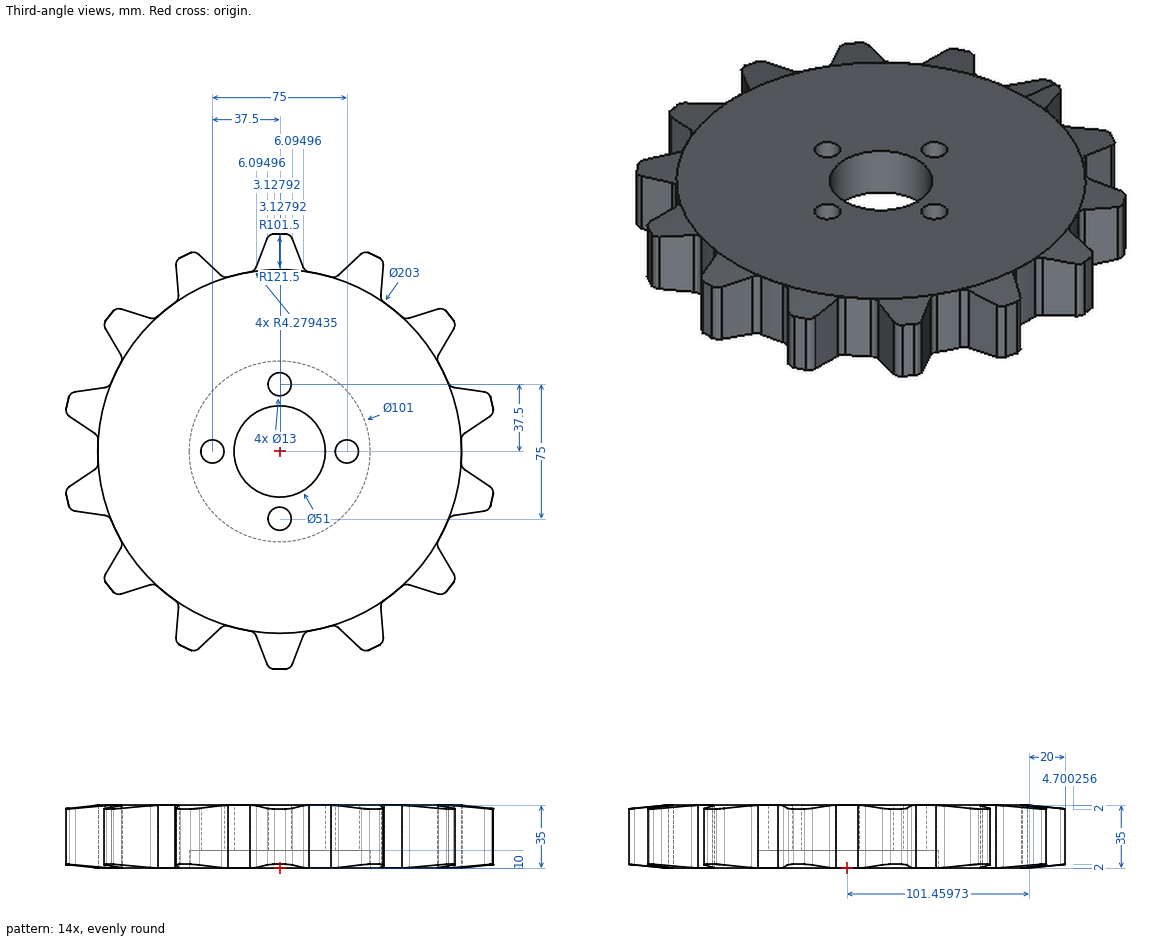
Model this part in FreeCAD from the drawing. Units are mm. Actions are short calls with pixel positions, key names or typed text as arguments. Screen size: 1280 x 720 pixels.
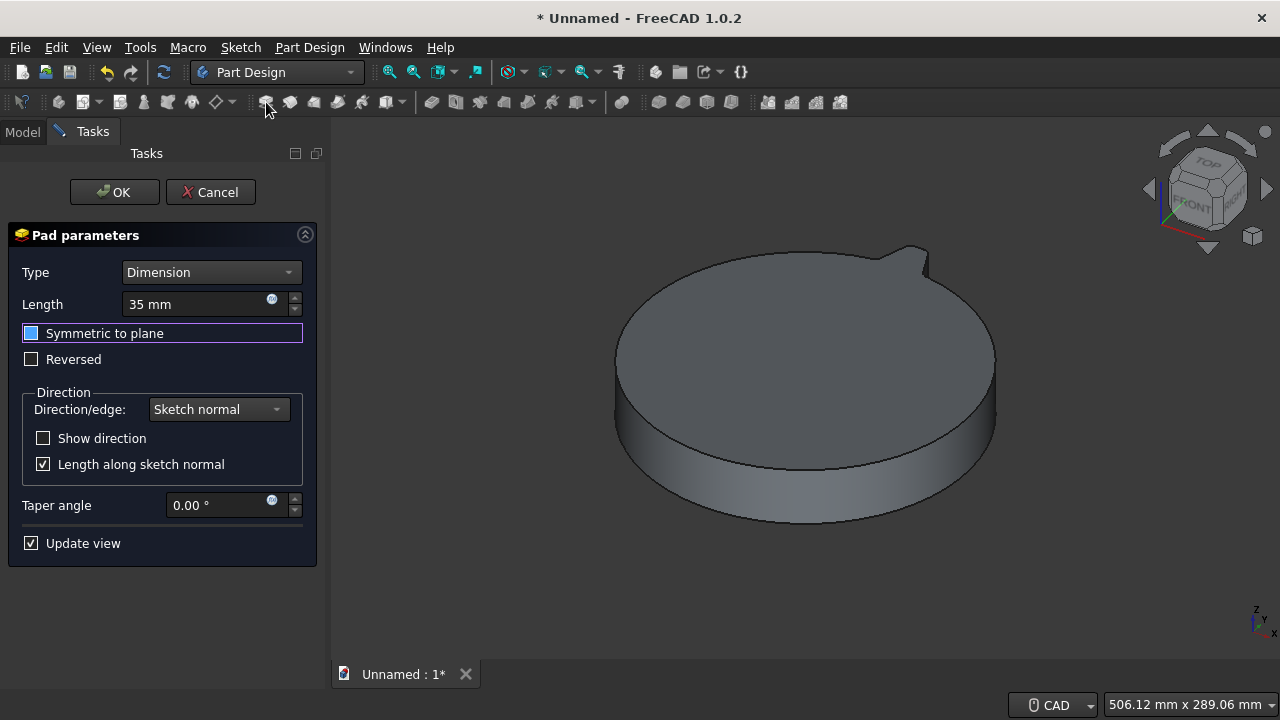
click(115, 192)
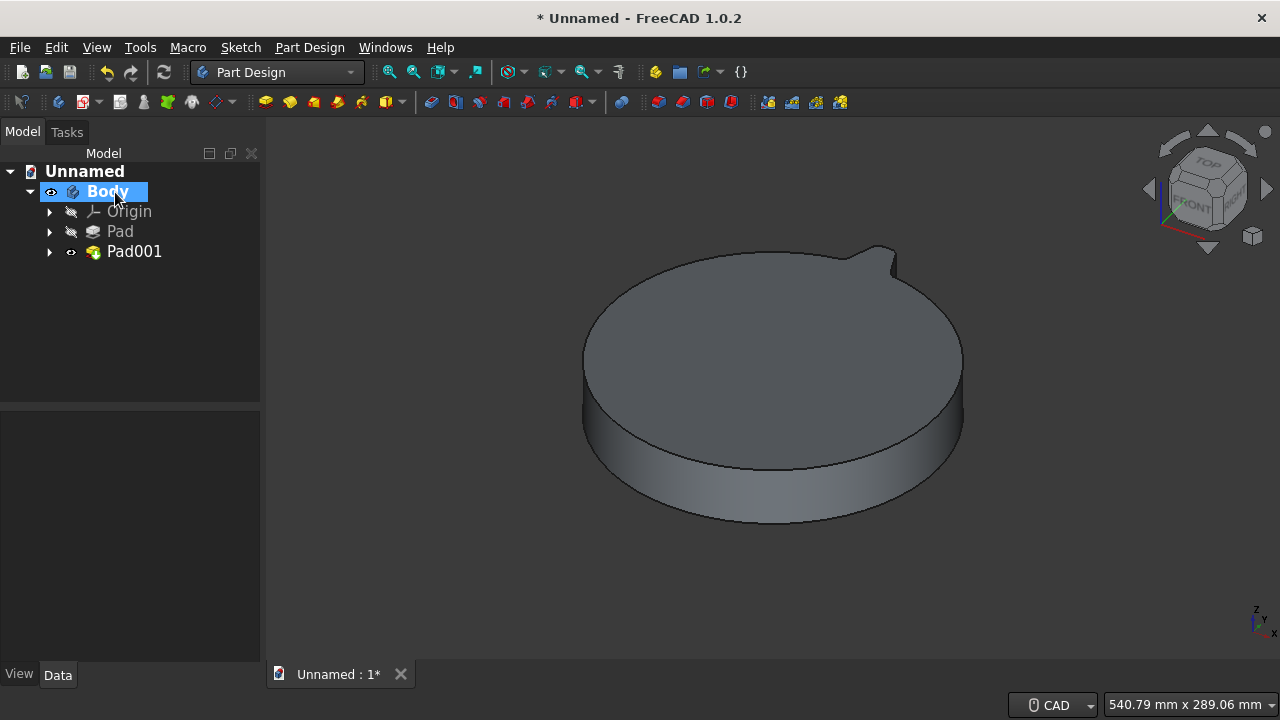
click(116, 252)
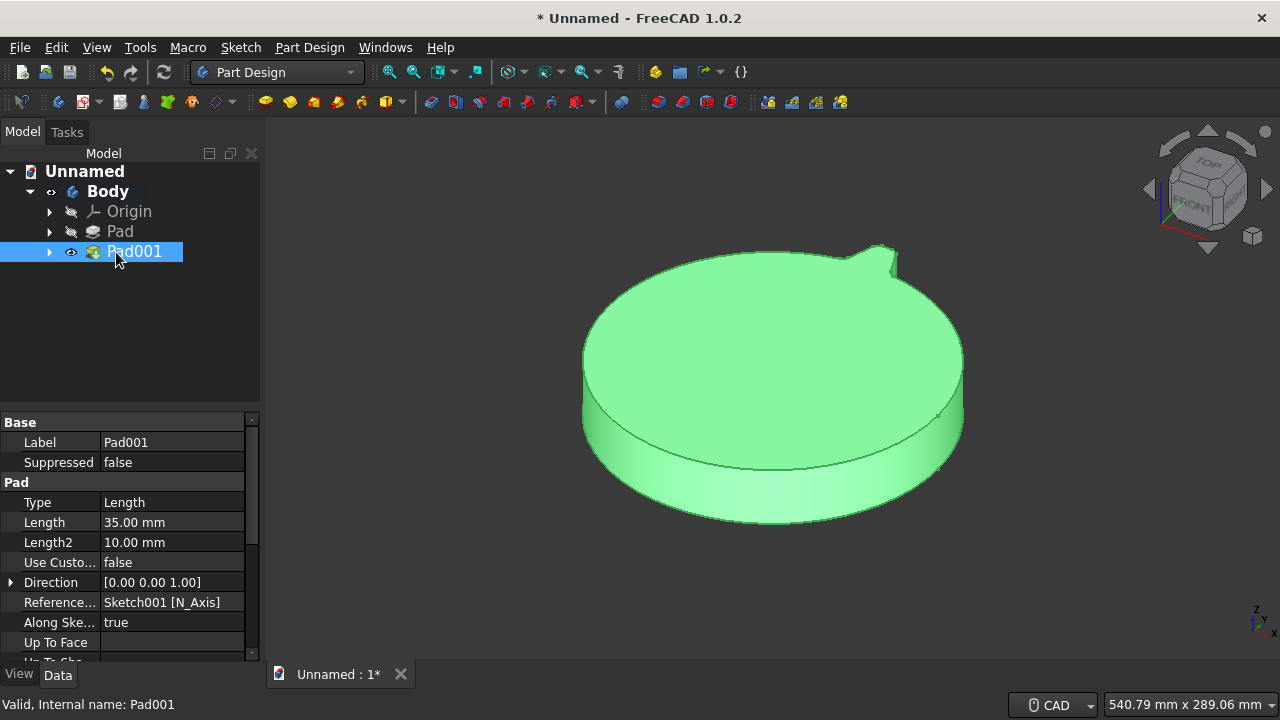
click(816, 102)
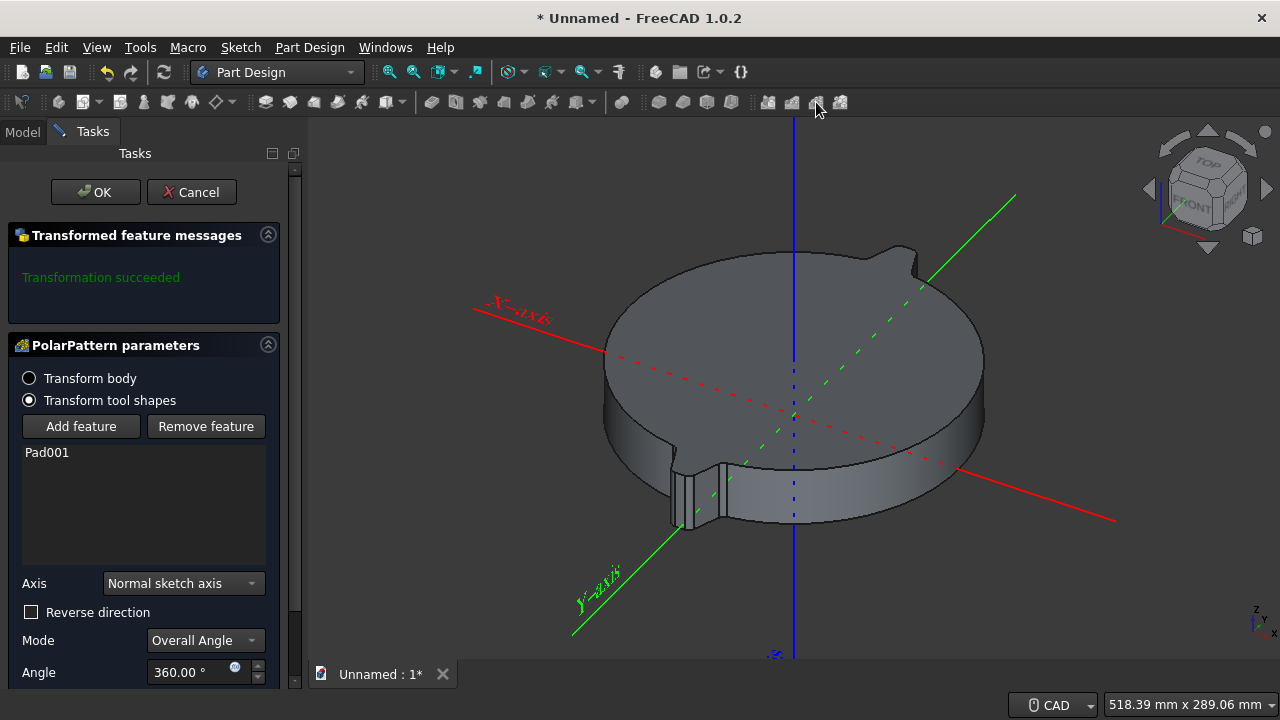
click(184, 584)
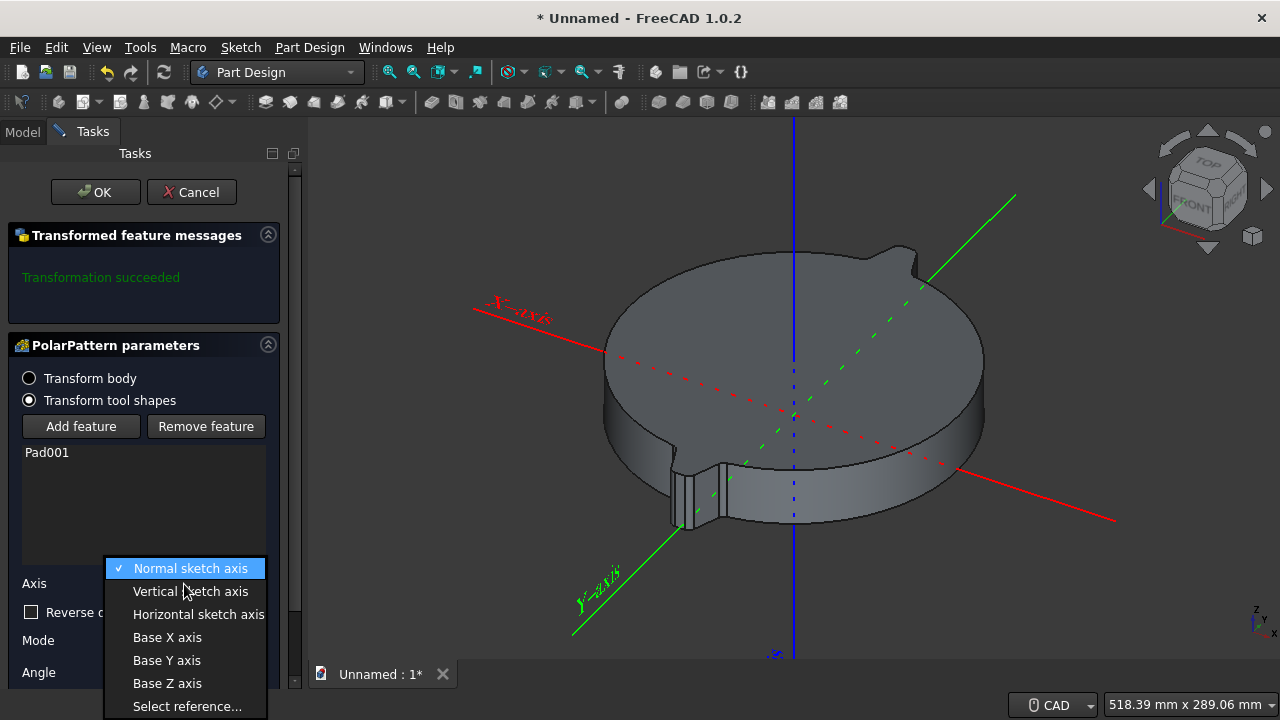
click(184, 684)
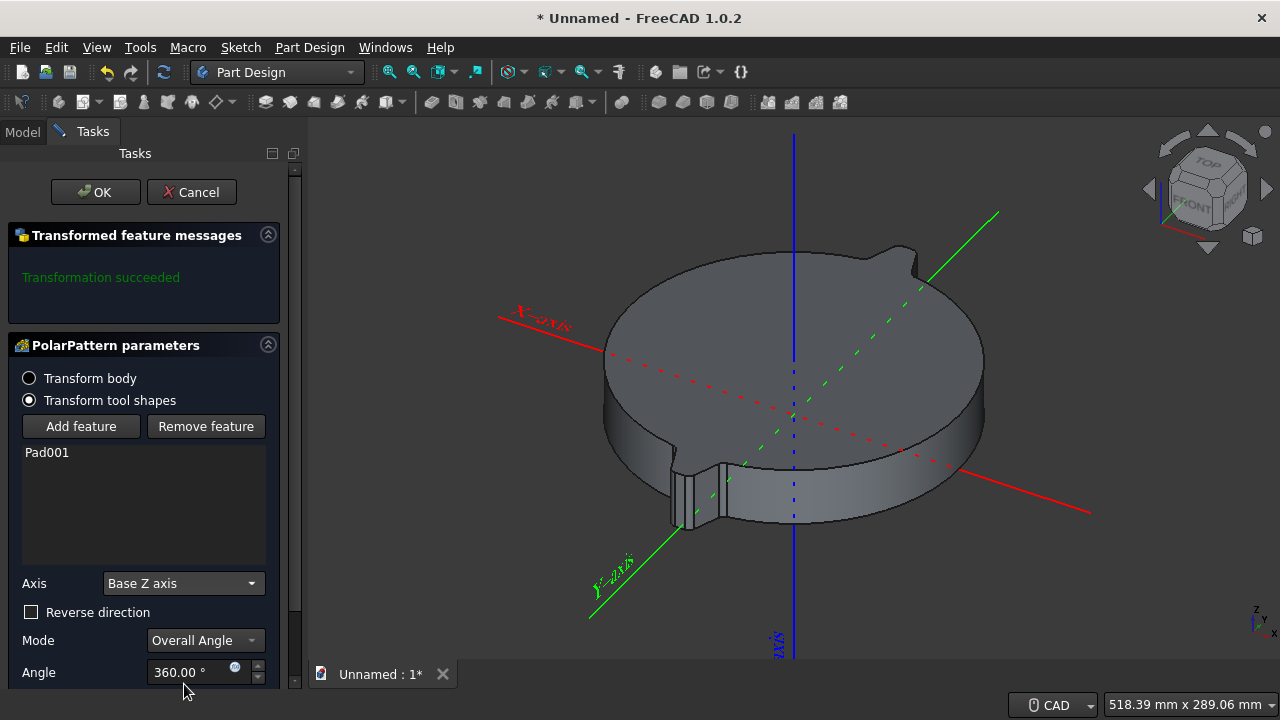
scroll(295, 426, down, 2)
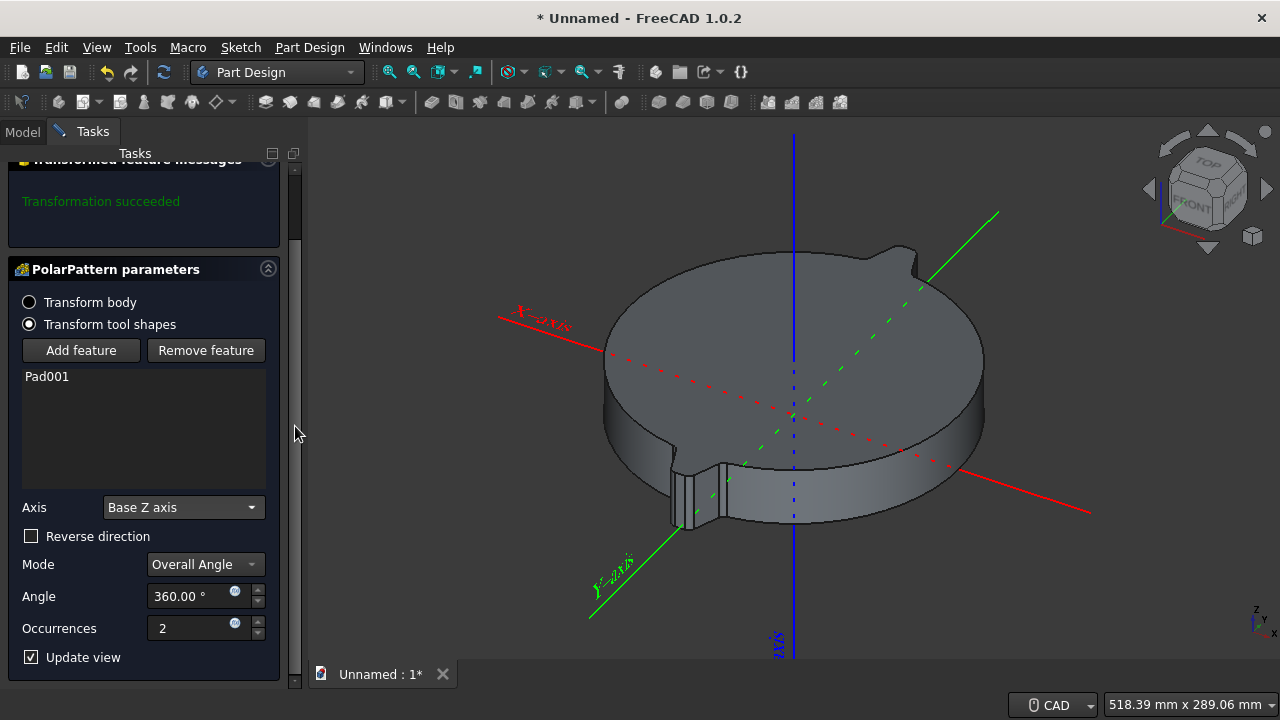
triple_click(198, 628)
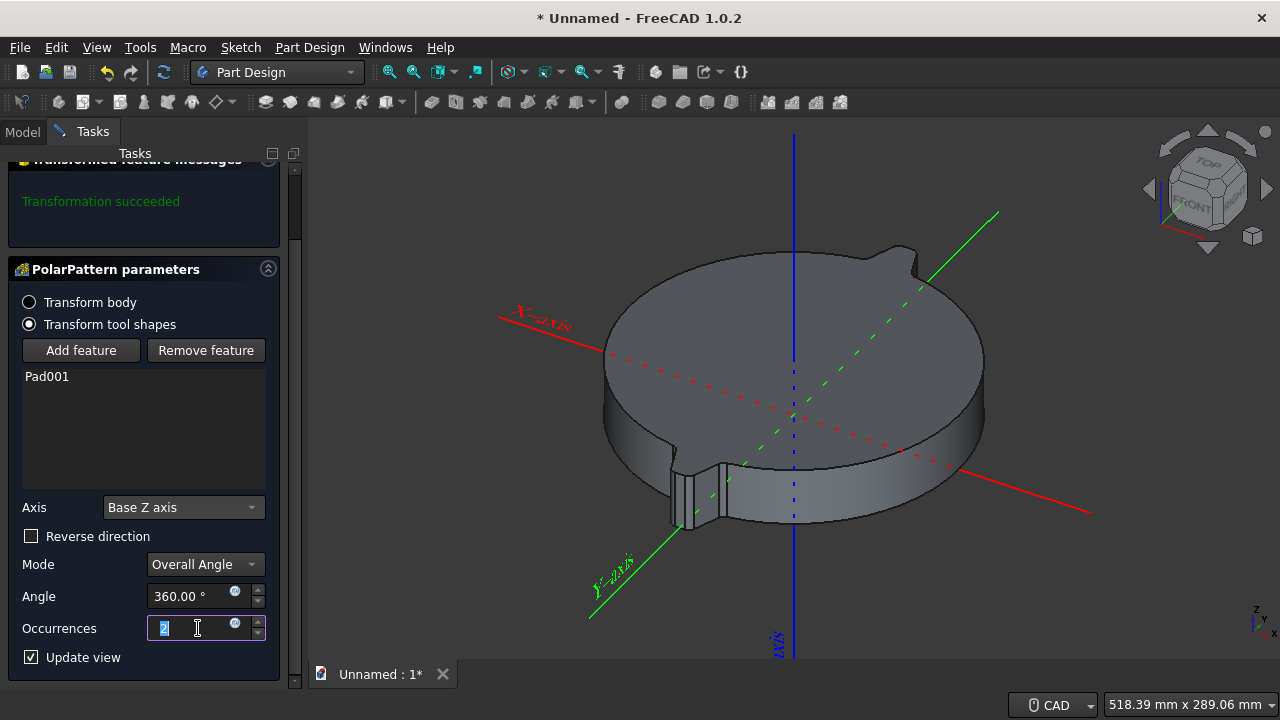
text(14)
key(Tab)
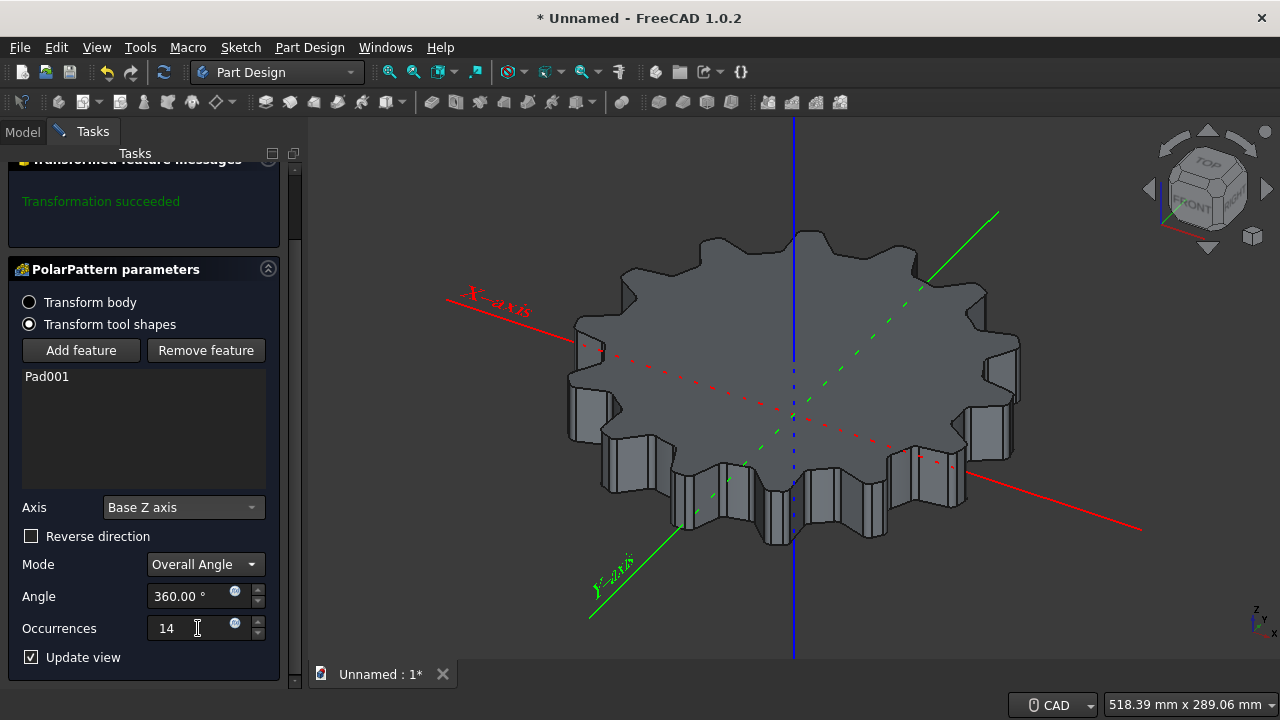
scroll(295, 426, up, 3)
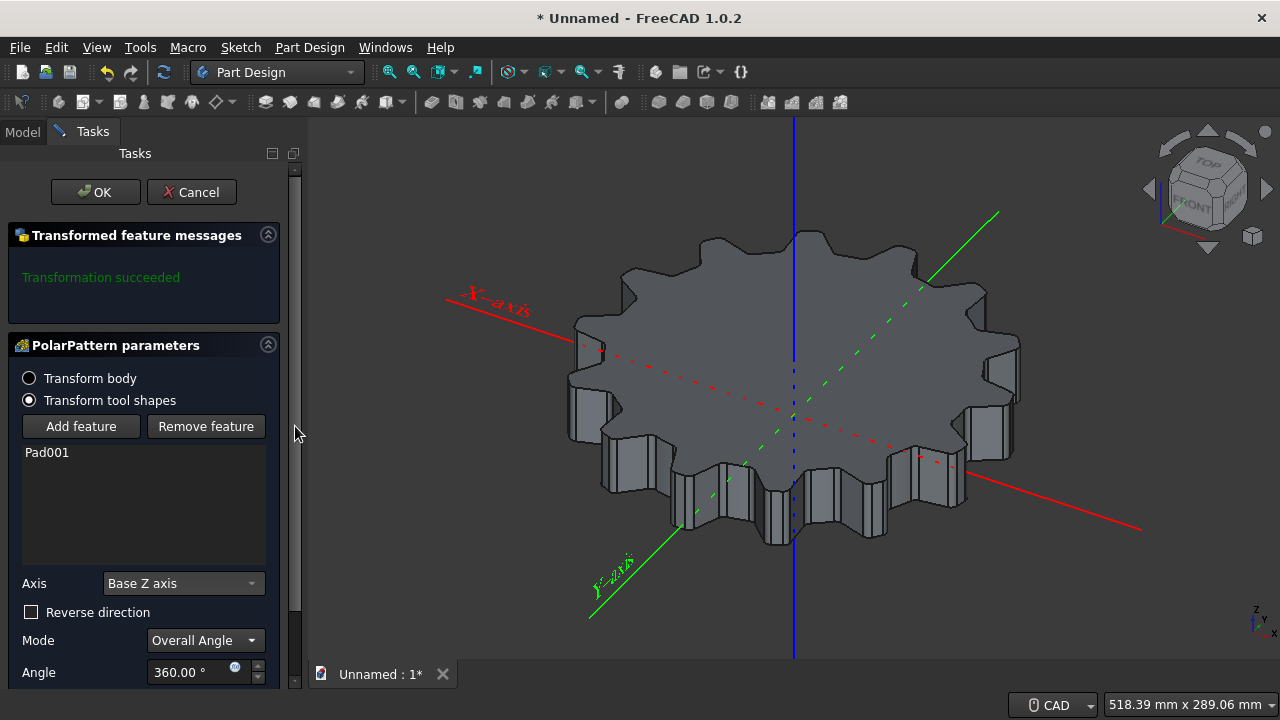
click(96, 192)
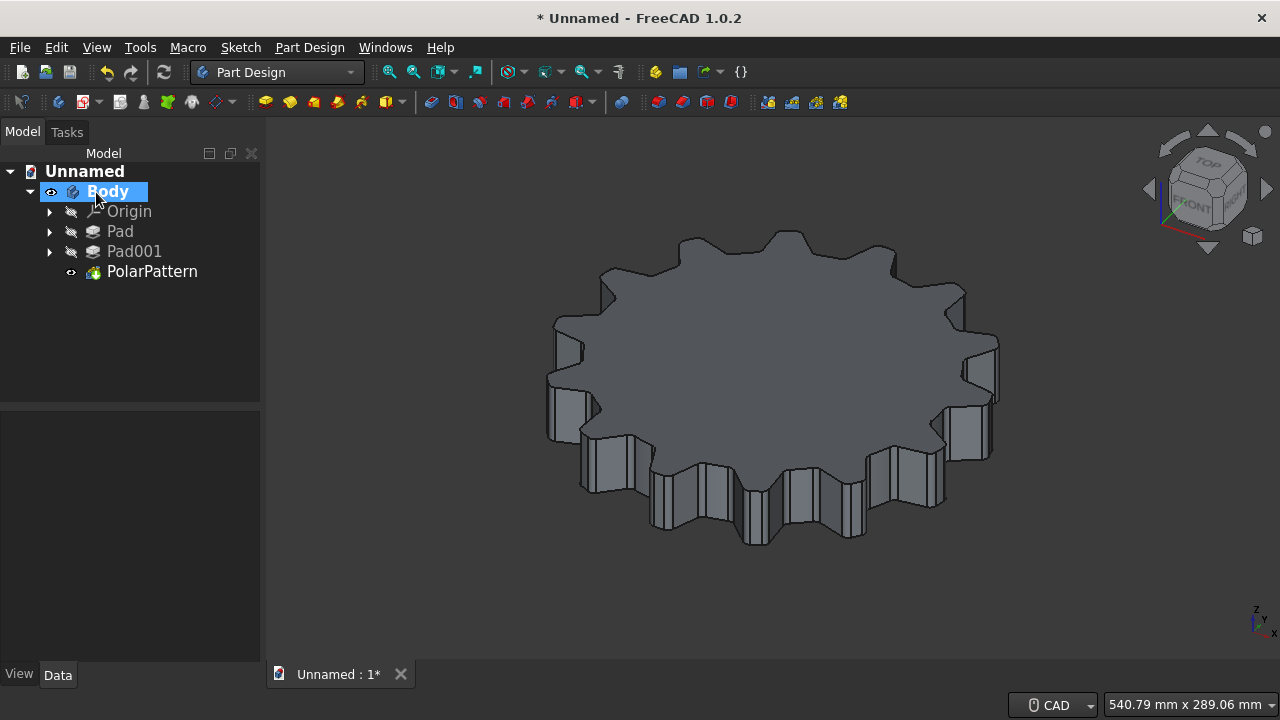
click(84, 102)